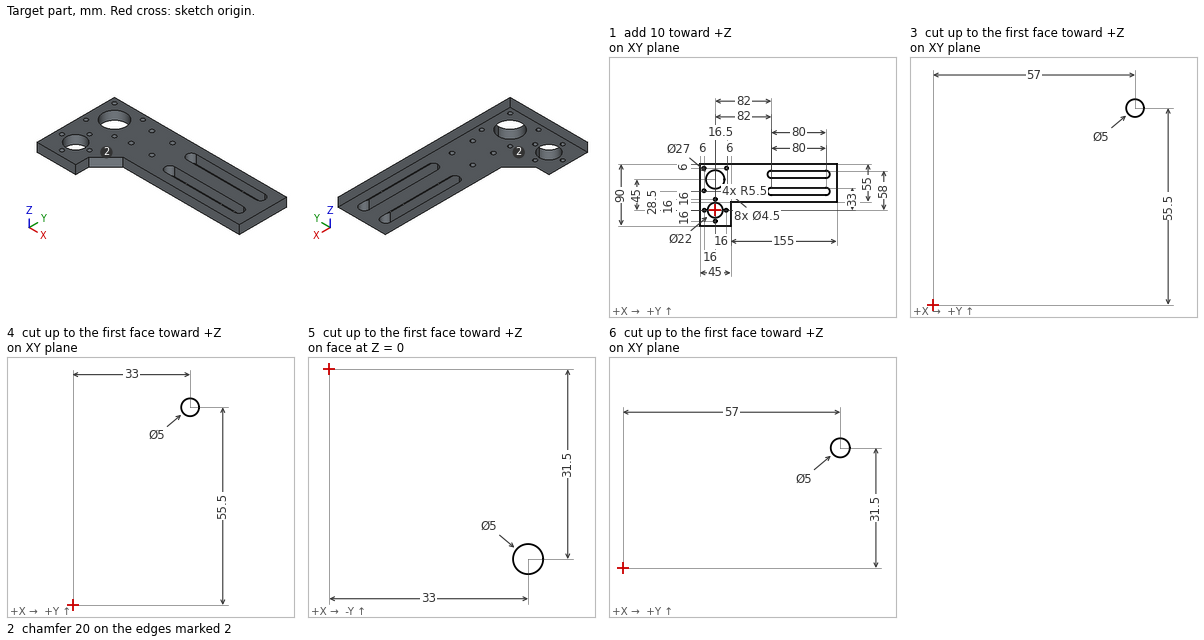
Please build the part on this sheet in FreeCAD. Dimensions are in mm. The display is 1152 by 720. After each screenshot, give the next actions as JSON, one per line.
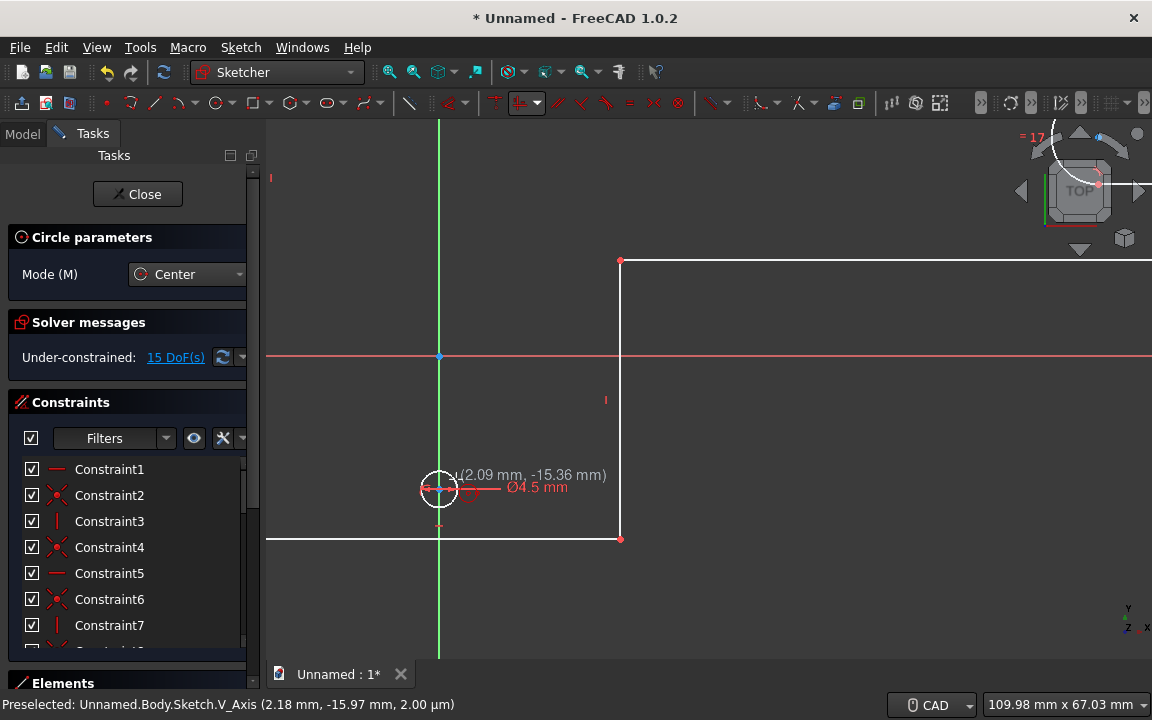
{"action": "scroll", "coordinate": [568, 356], "scroll_direction": "up", "scroll_amount": 2}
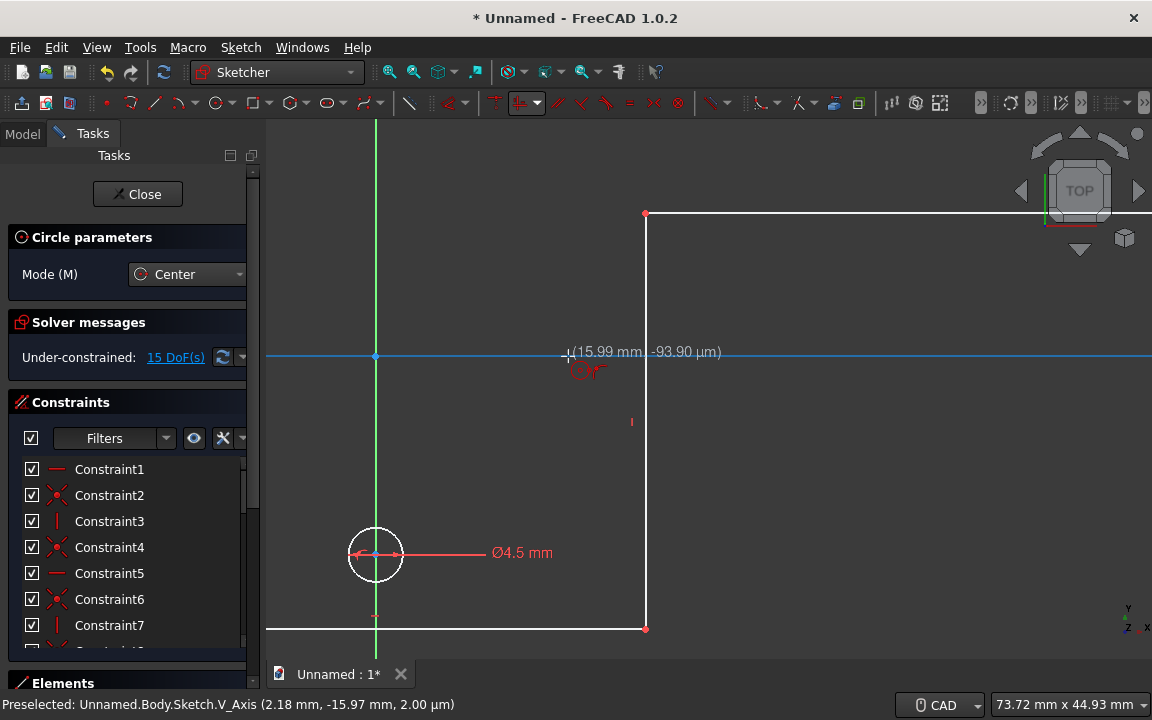
{"action": "scroll", "coordinate": [472, 466], "scroll_direction": "down", "scroll_amount": 8}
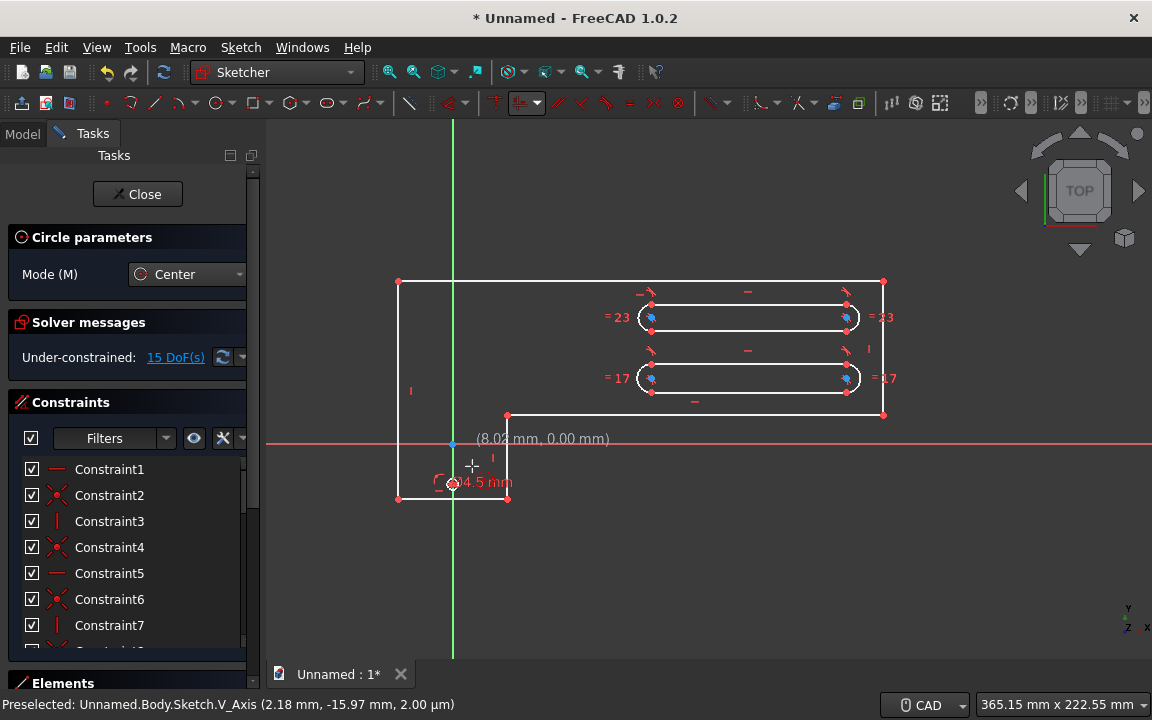
{"action": "left_click", "coordinate": [492, 444]}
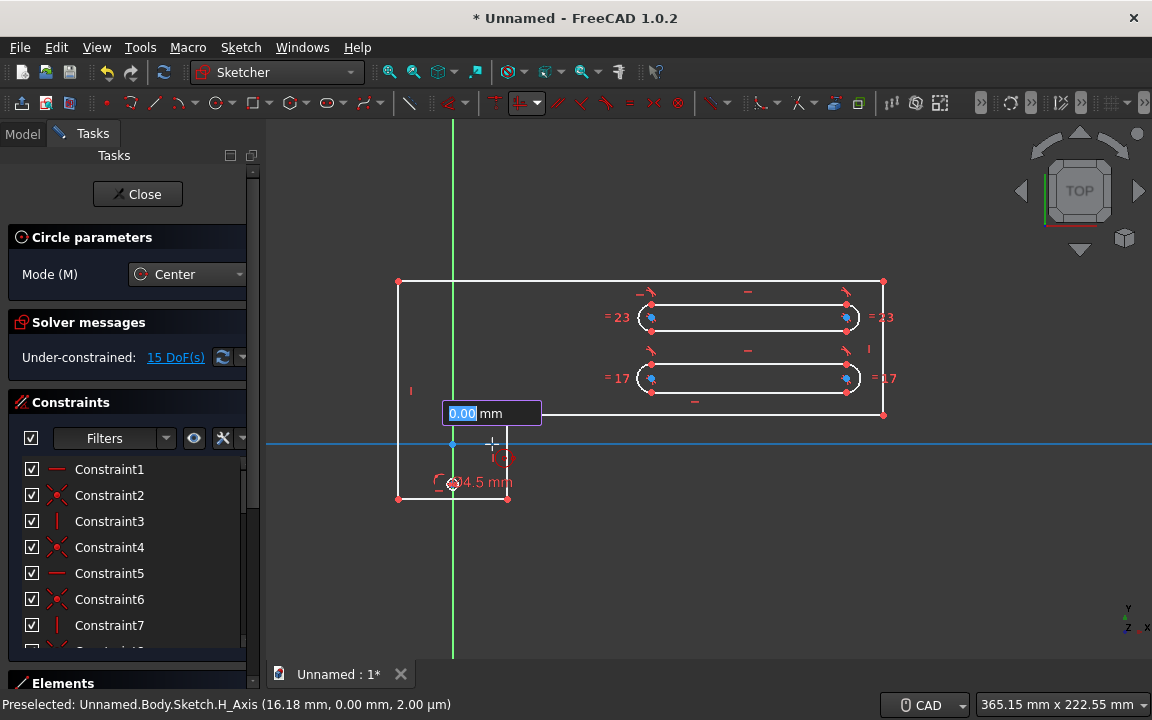
{"action": "scroll", "coordinate": [490, 449], "scroll_direction": "up", "scroll_amount": 6}
{"action": "mouse_move", "coordinate": [488, 449]}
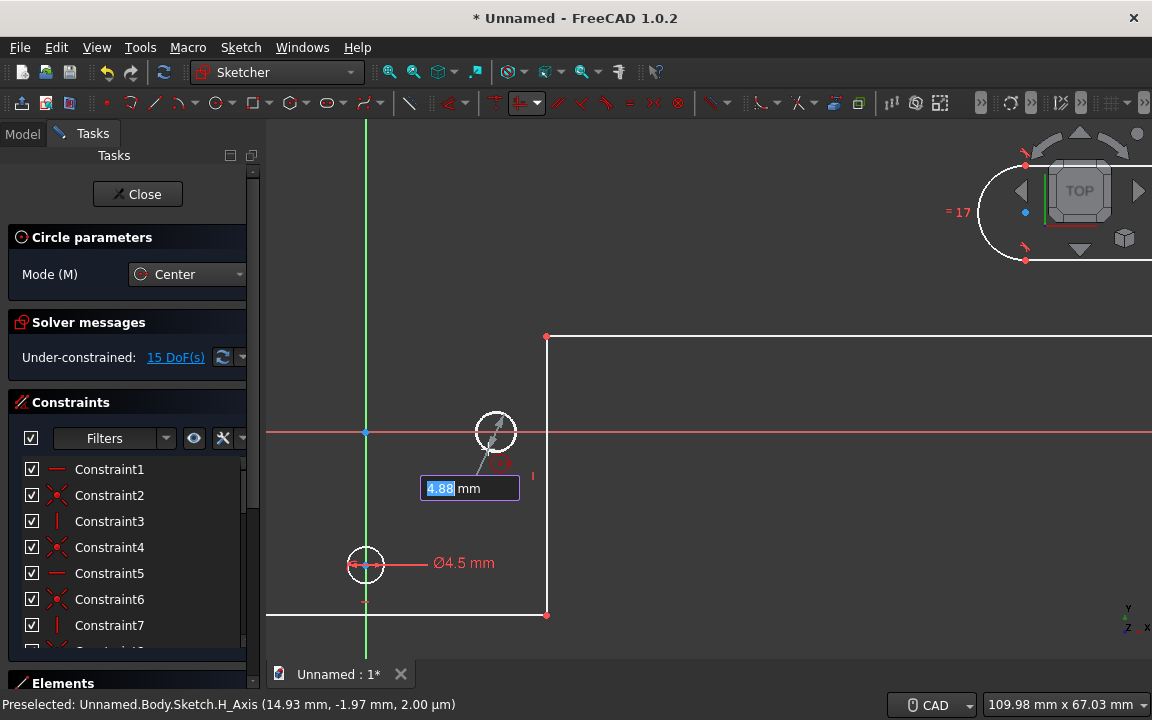
{"action": "type", "text": "4.5"}
{"action": "key", "text": "Return"}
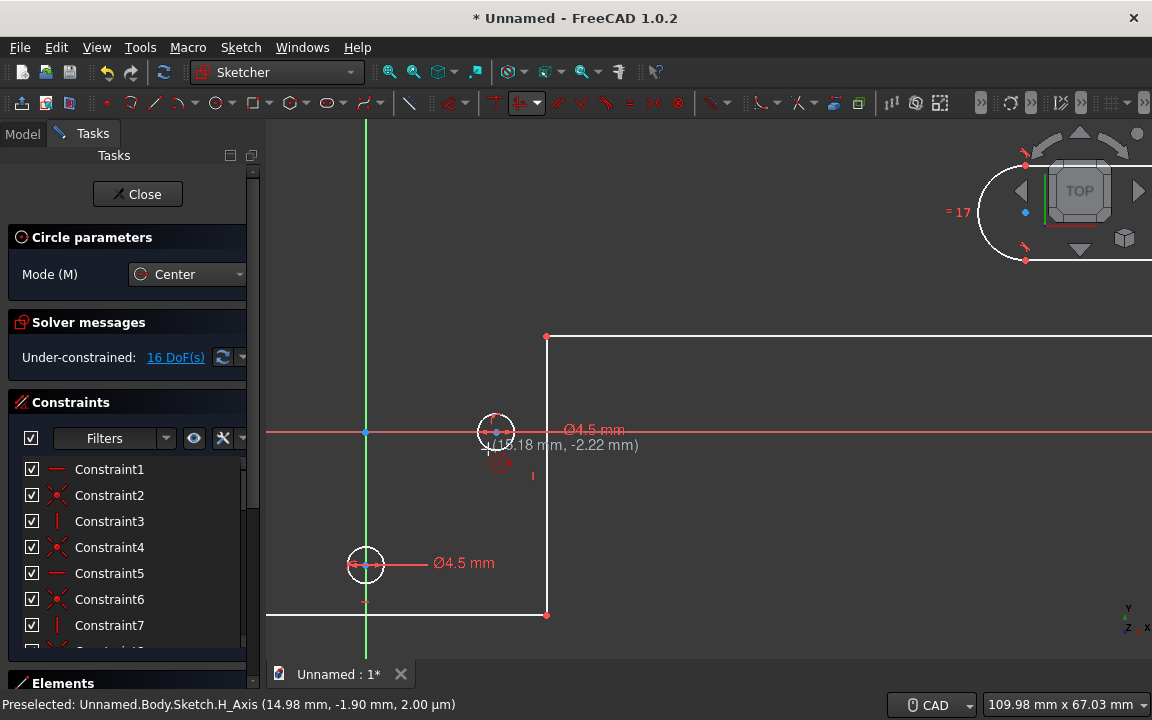
{"action": "left_click", "coordinate": [366, 432]}
{"action": "mouse_move", "coordinate": [428, 369]}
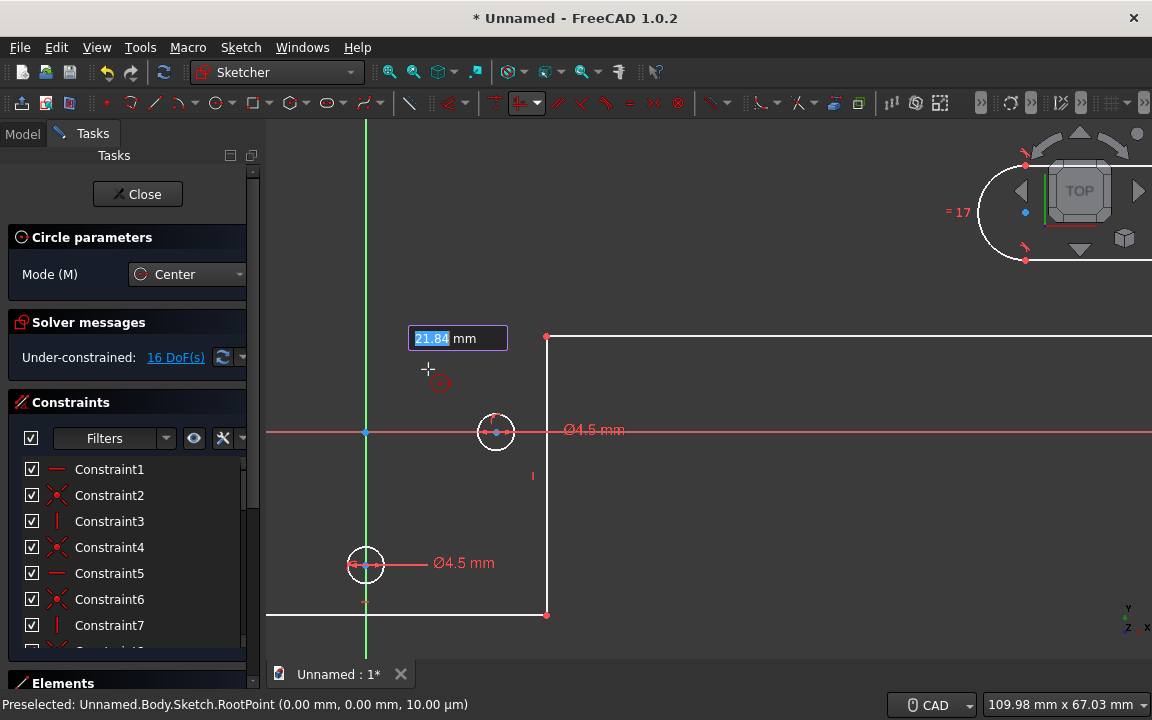
{"action": "type", "text": "22"}
{"action": "key", "text": "Return"}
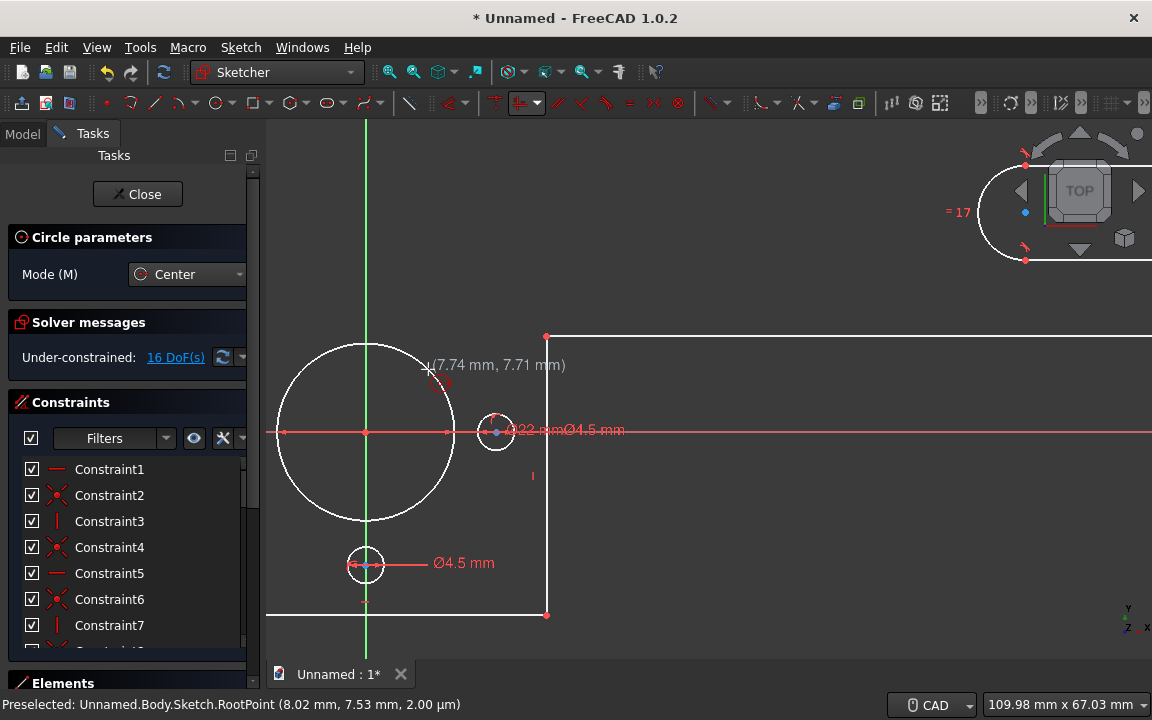
{"action": "scroll", "coordinate": [490, 449], "scroll_direction": "down", "scroll_amount": 6}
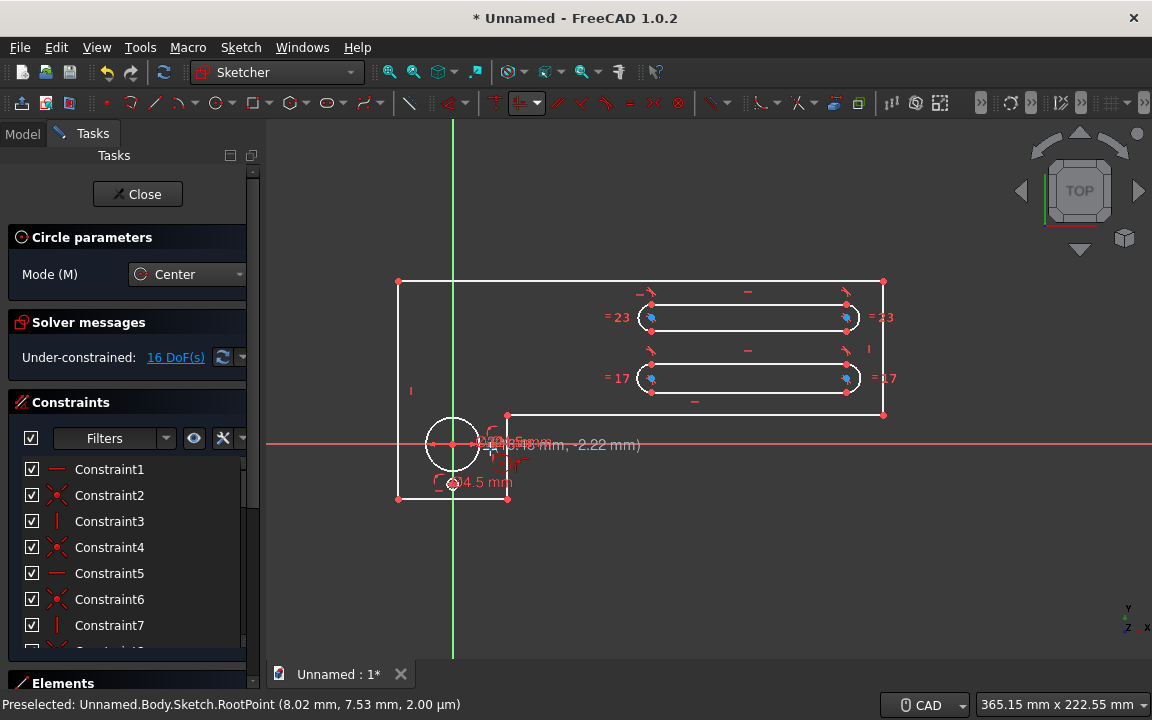
{"action": "scroll", "coordinate": [414, 444], "scroll_direction": "up", "scroll_amount": 8}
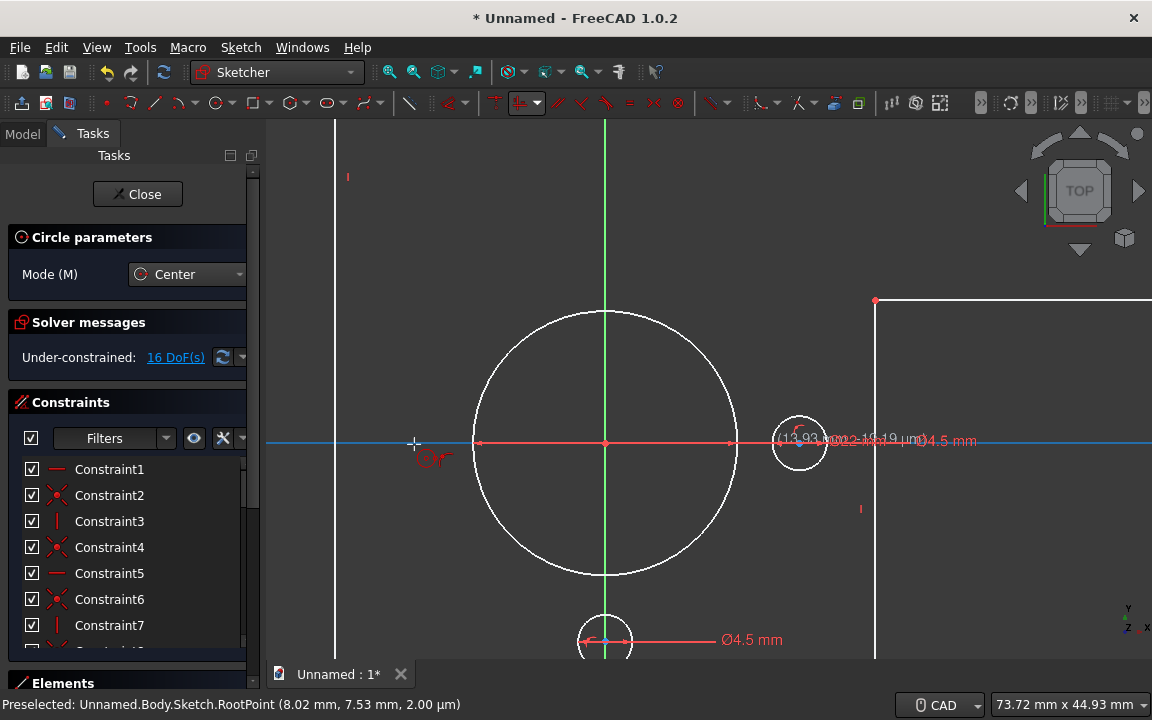
{"action": "scroll", "coordinate": [414, 444], "scroll_direction": "down", "scroll_amount": 8}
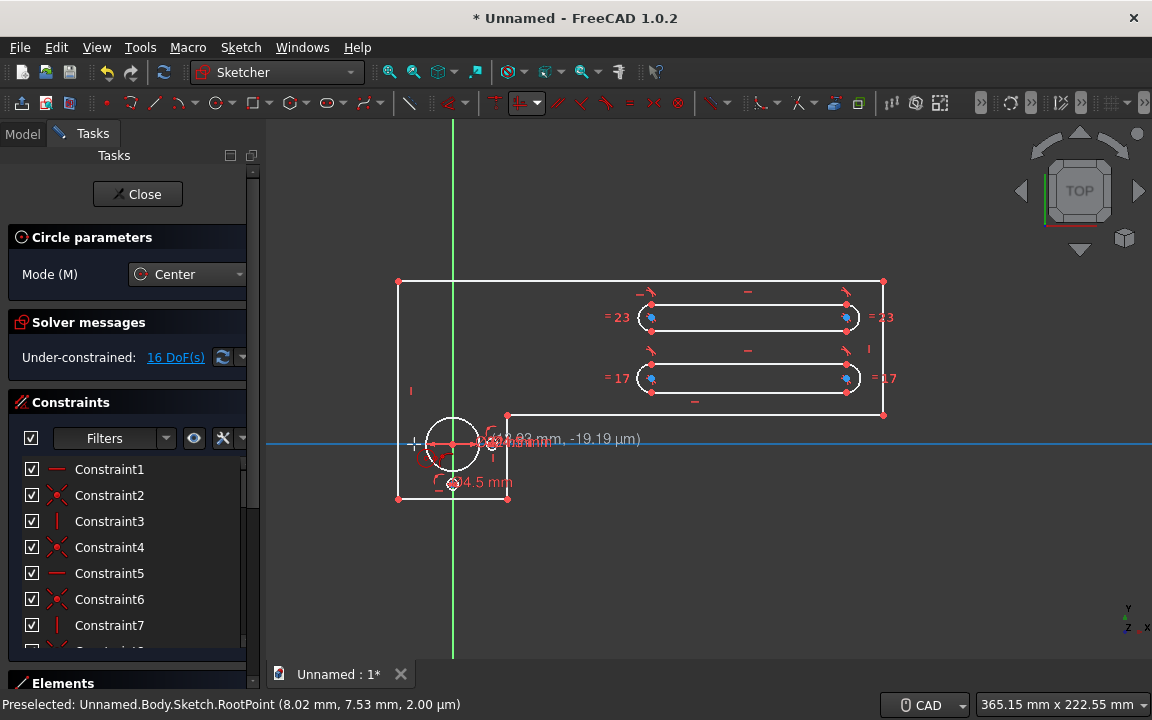
{"action": "scroll", "coordinate": [414, 444], "scroll_direction": "up", "scroll_amount": 2}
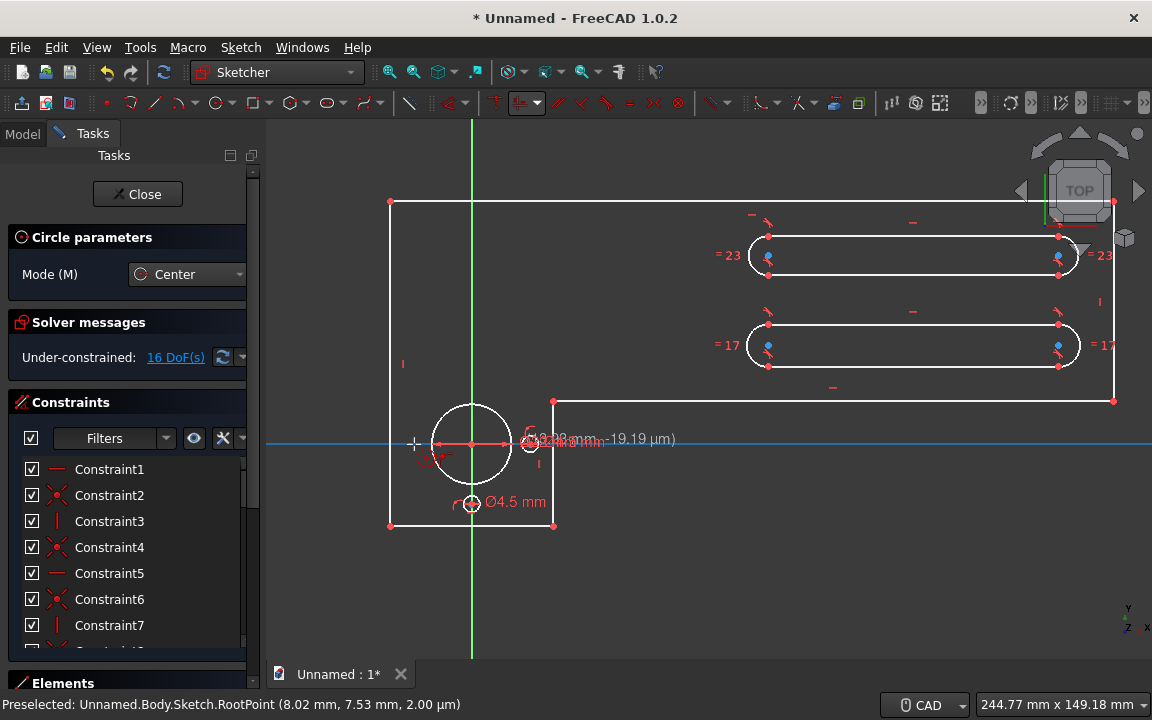
{"action": "left_click", "coordinate": [414, 444]}